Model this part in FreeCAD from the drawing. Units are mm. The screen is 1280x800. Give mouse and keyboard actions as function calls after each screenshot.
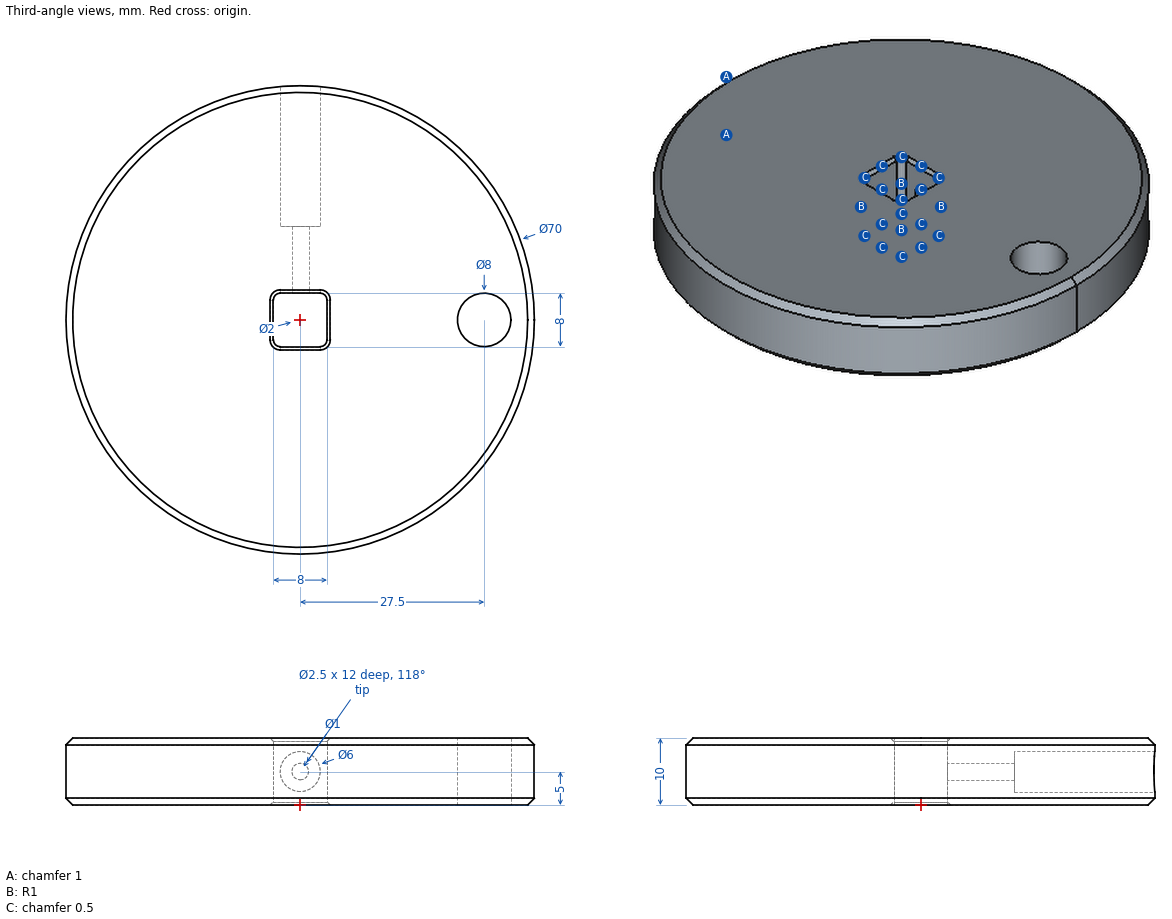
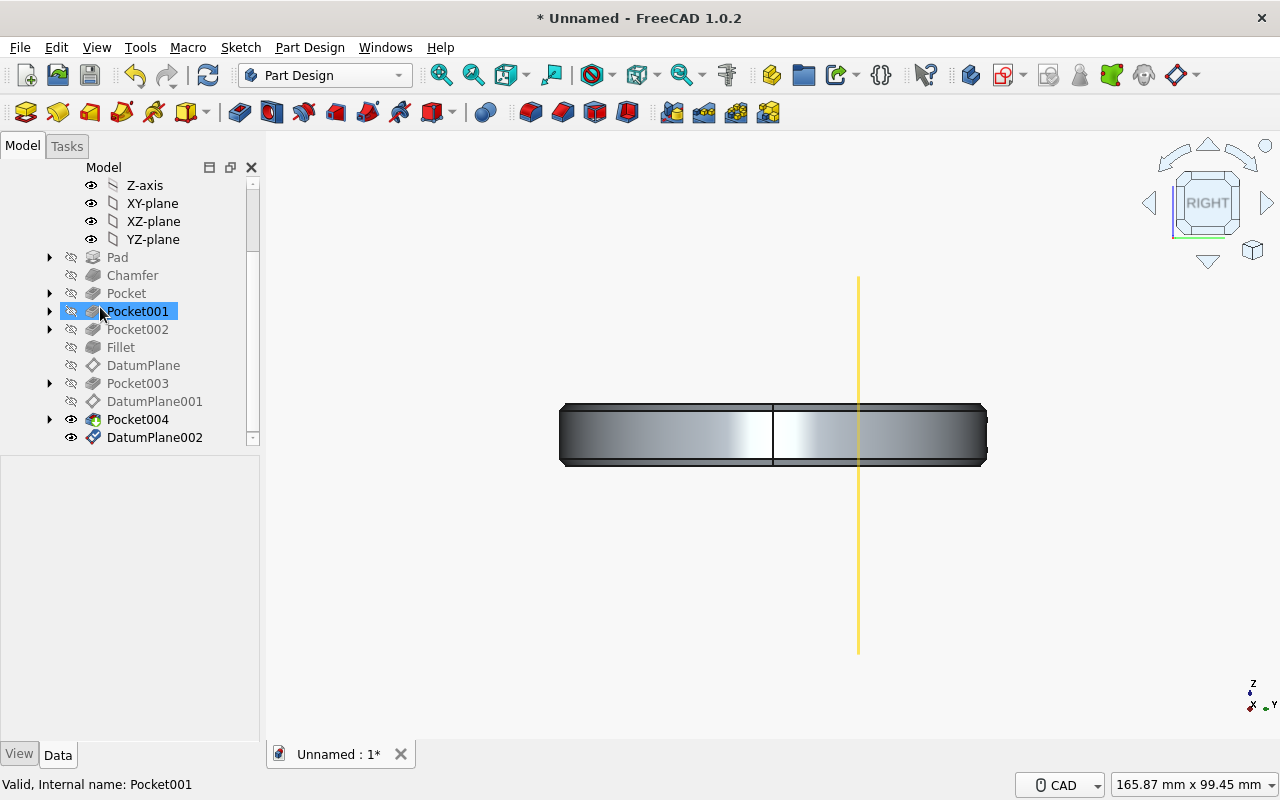
click(116, 437)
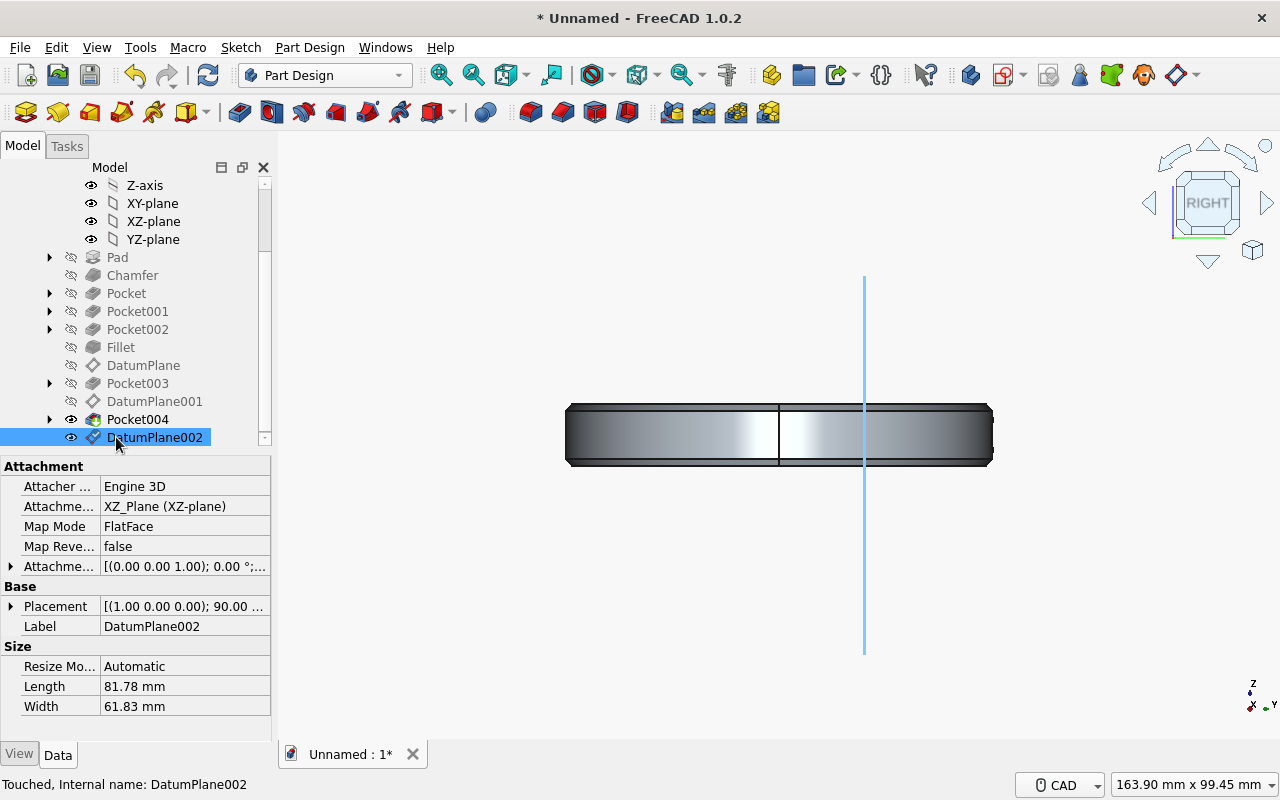
click(1004, 76)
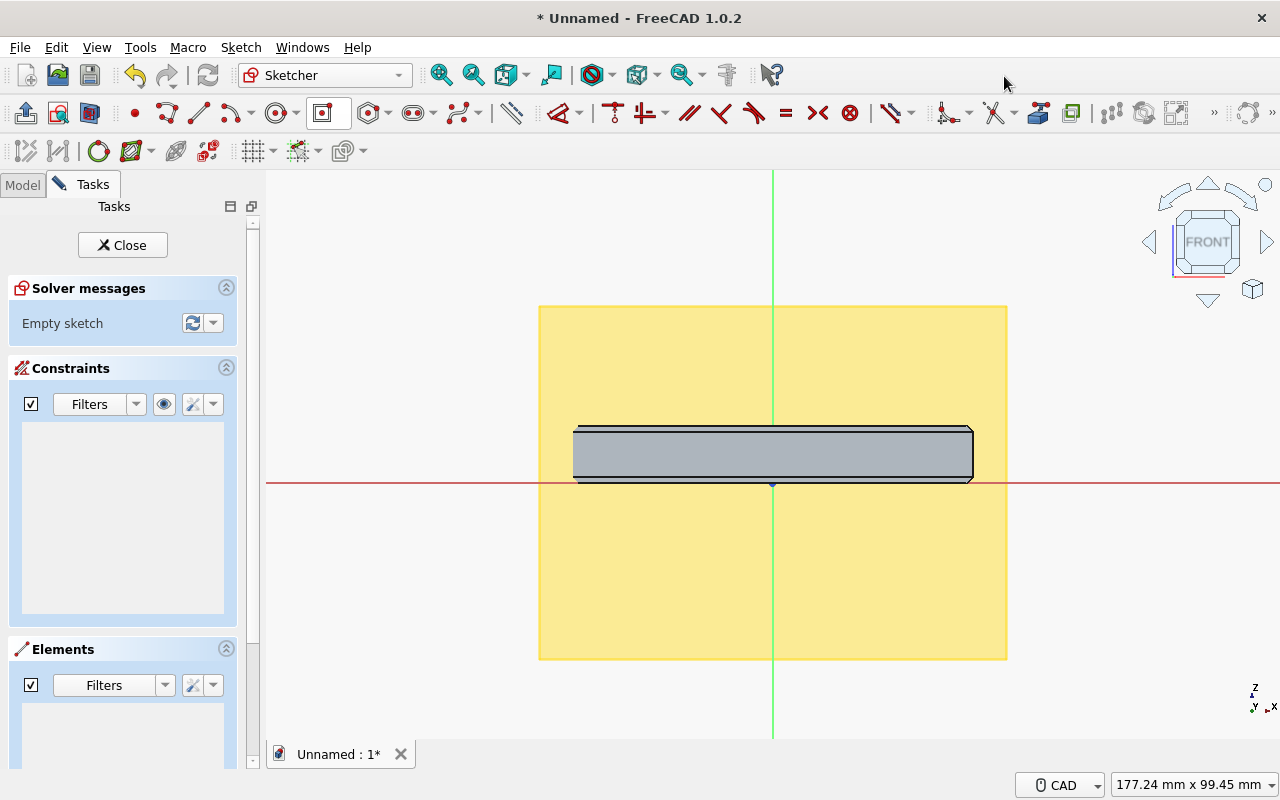
key(q)
key(s)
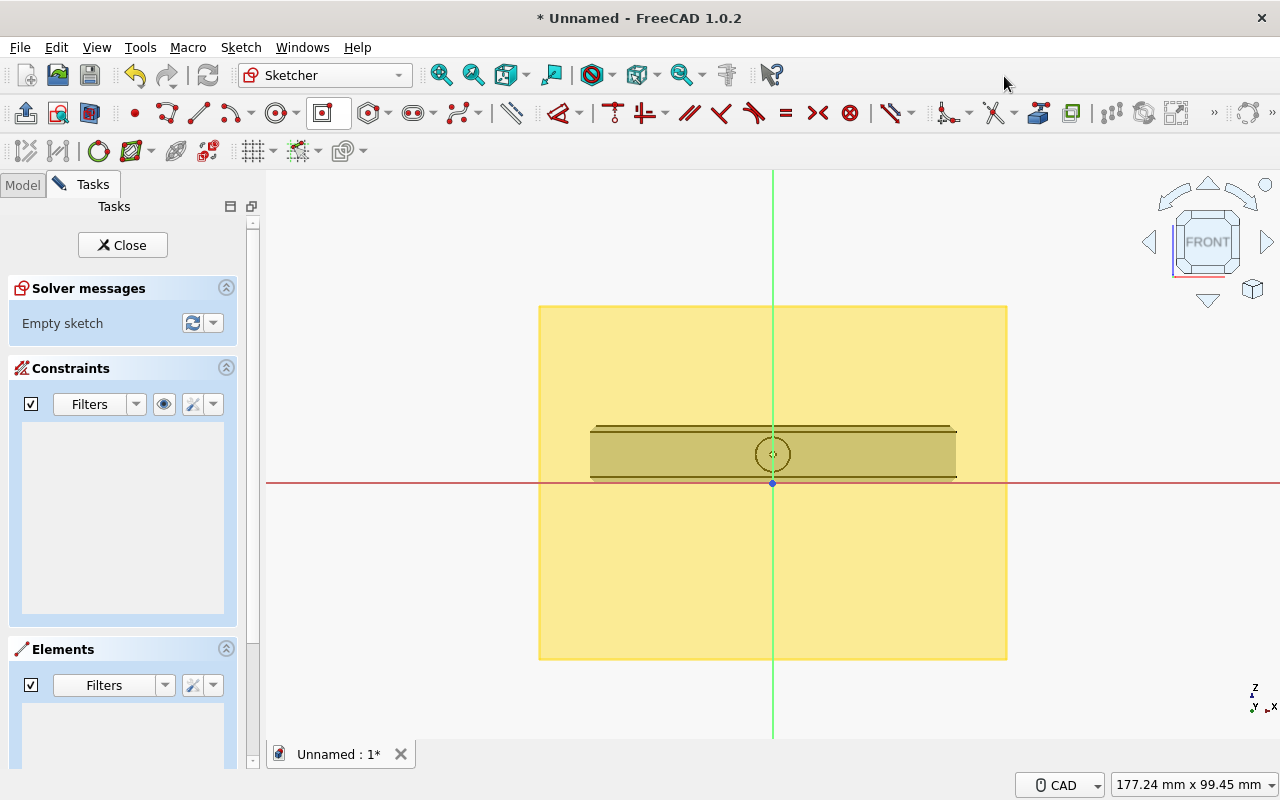
scroll(776, 455, up, 15)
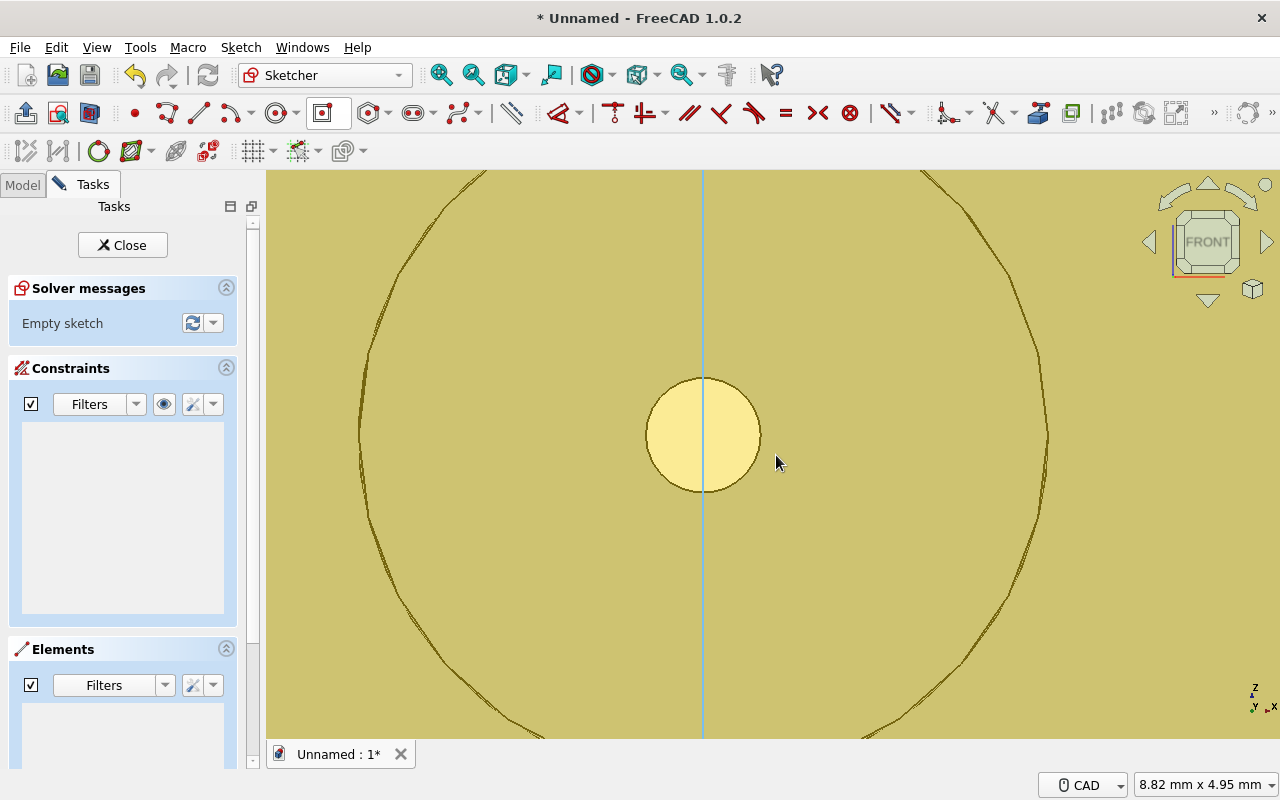
click(276, 114)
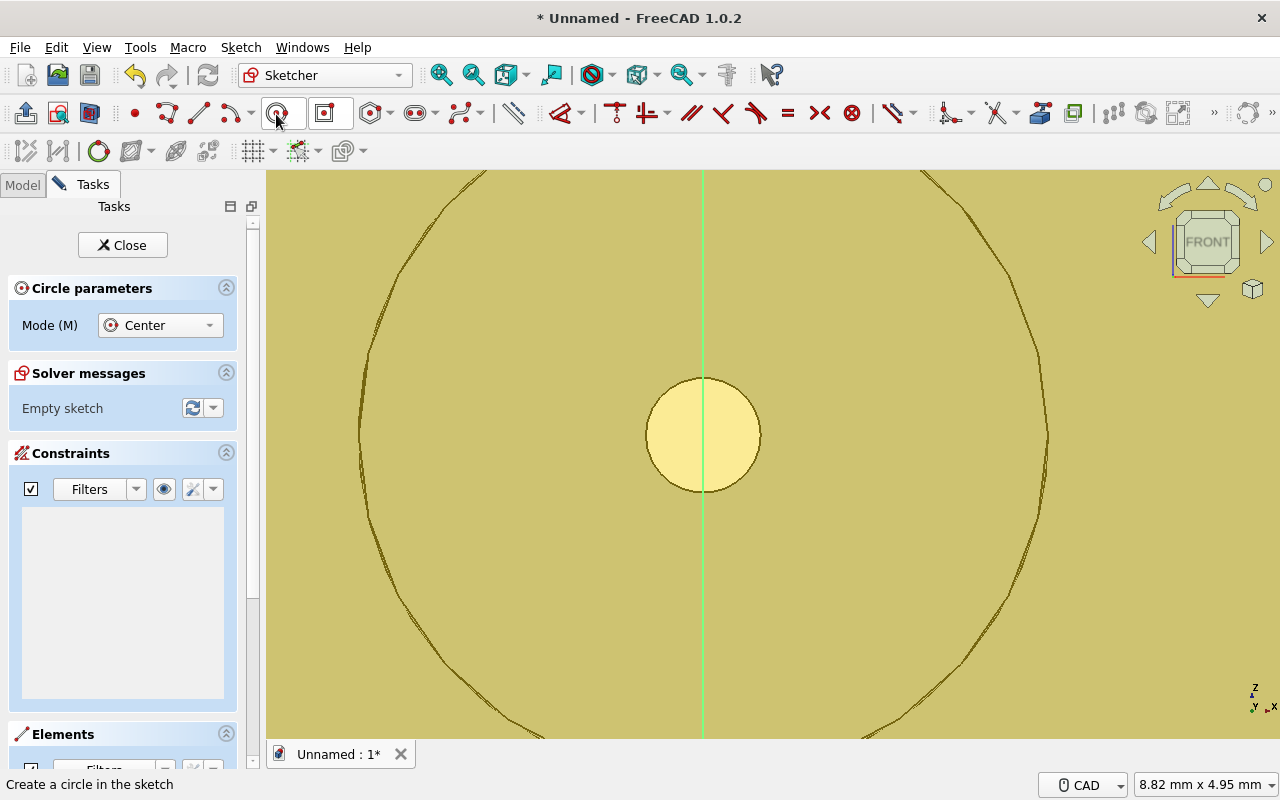
click(703, 435)
click(805, 334)
key(Escape)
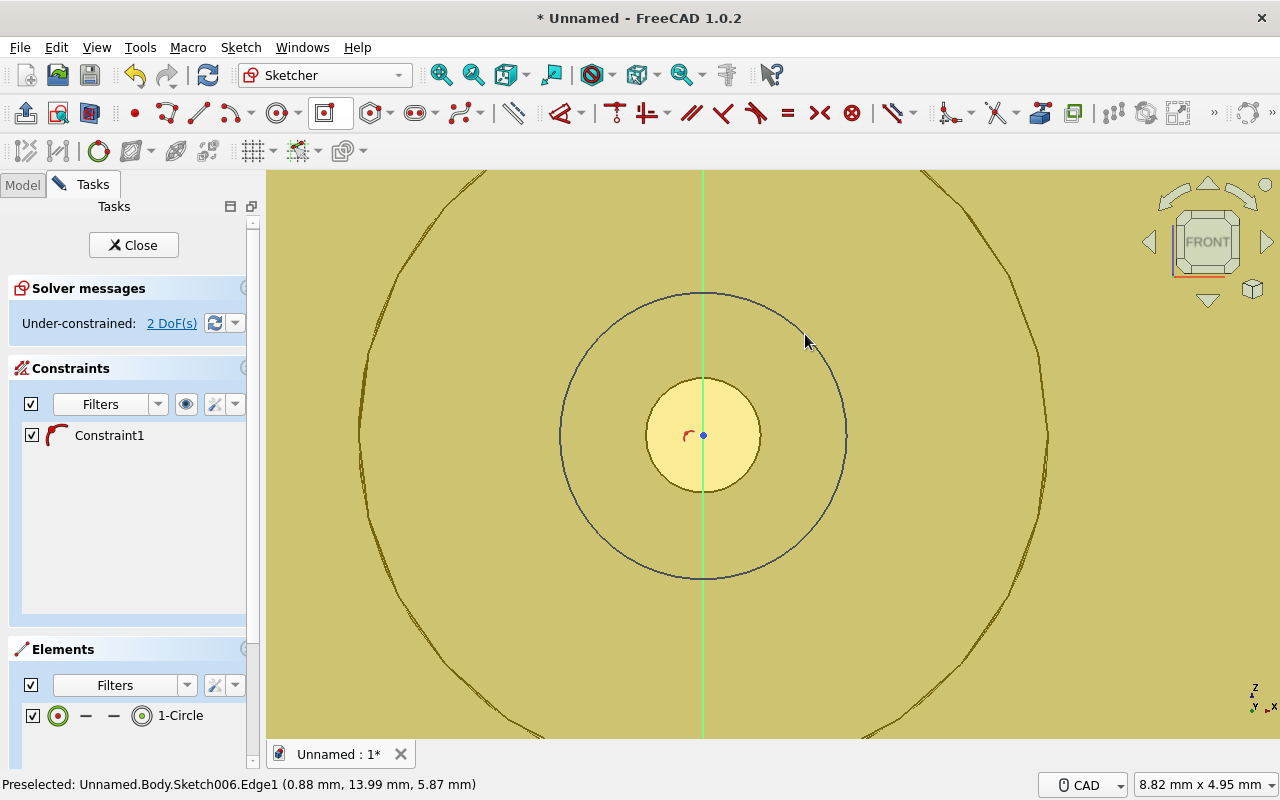
key(d)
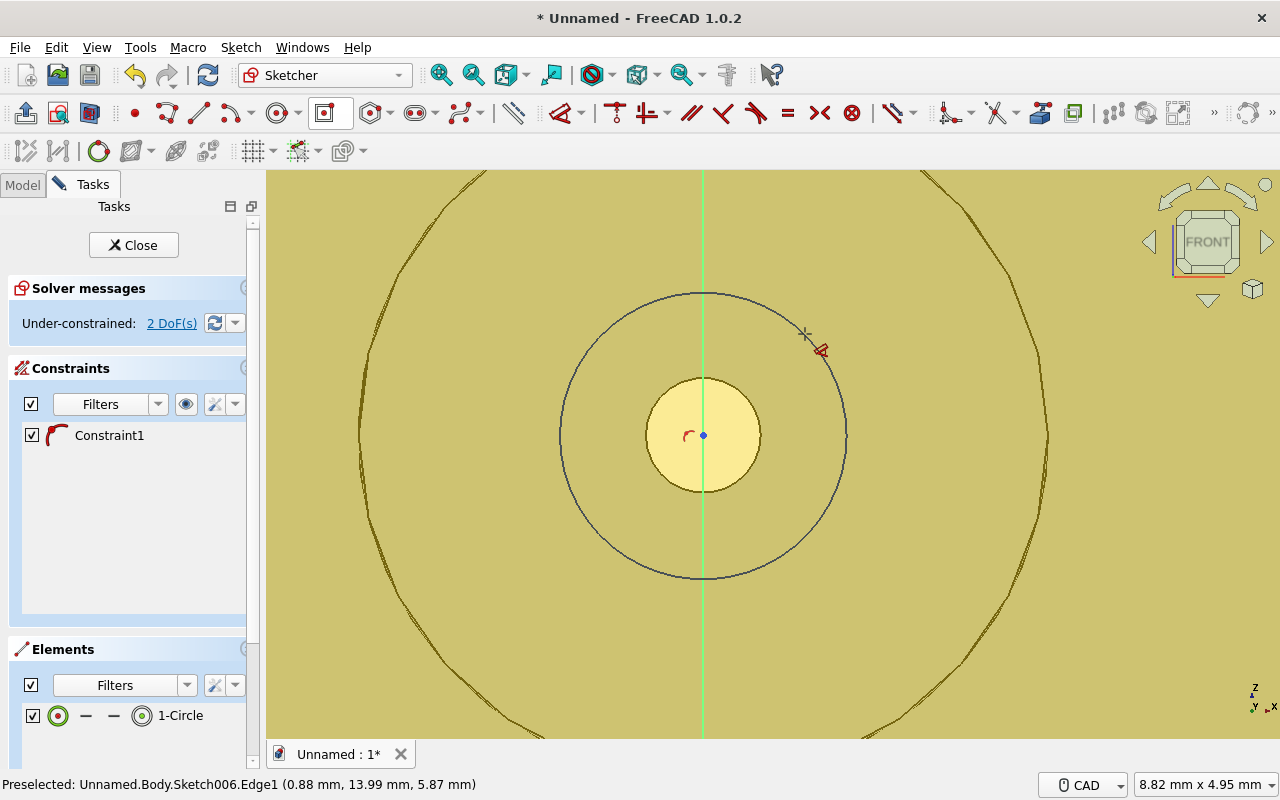
click(804, 334)
click(826, 311)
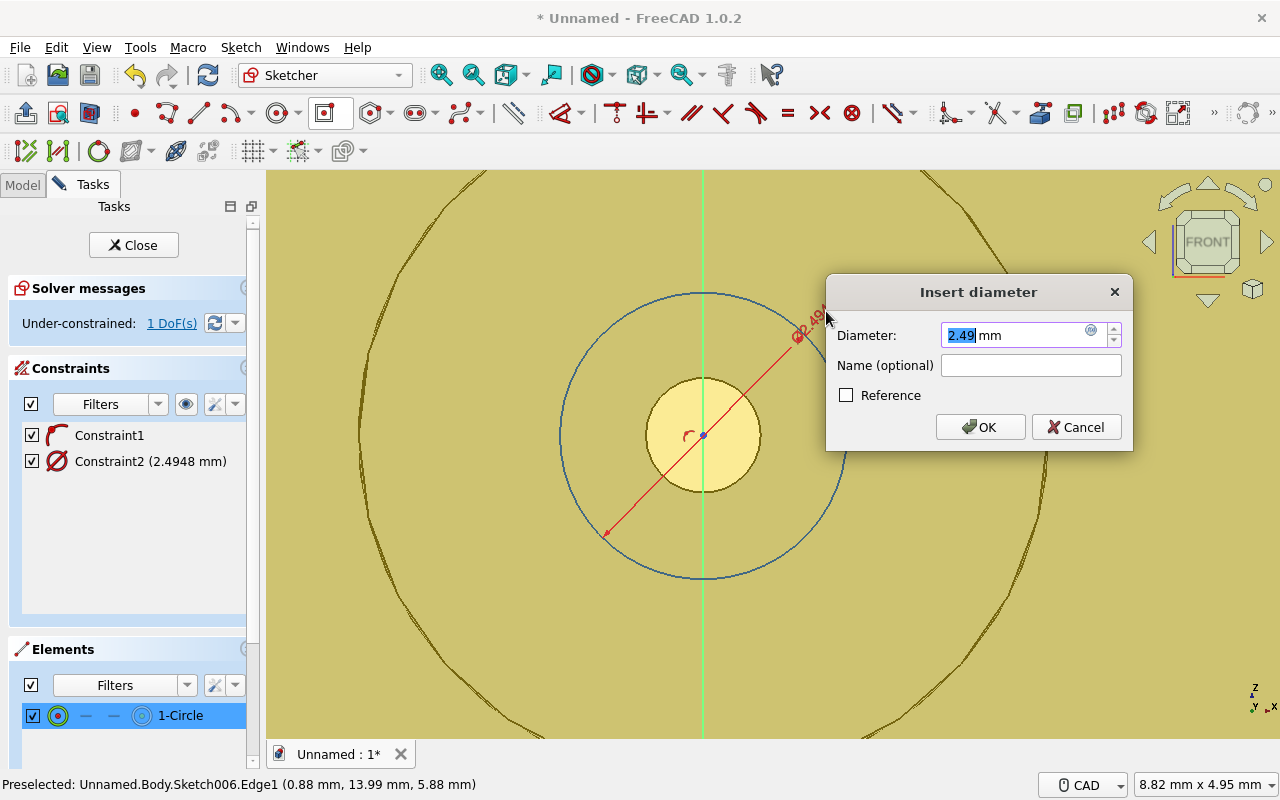
text(2.5)
key(Return)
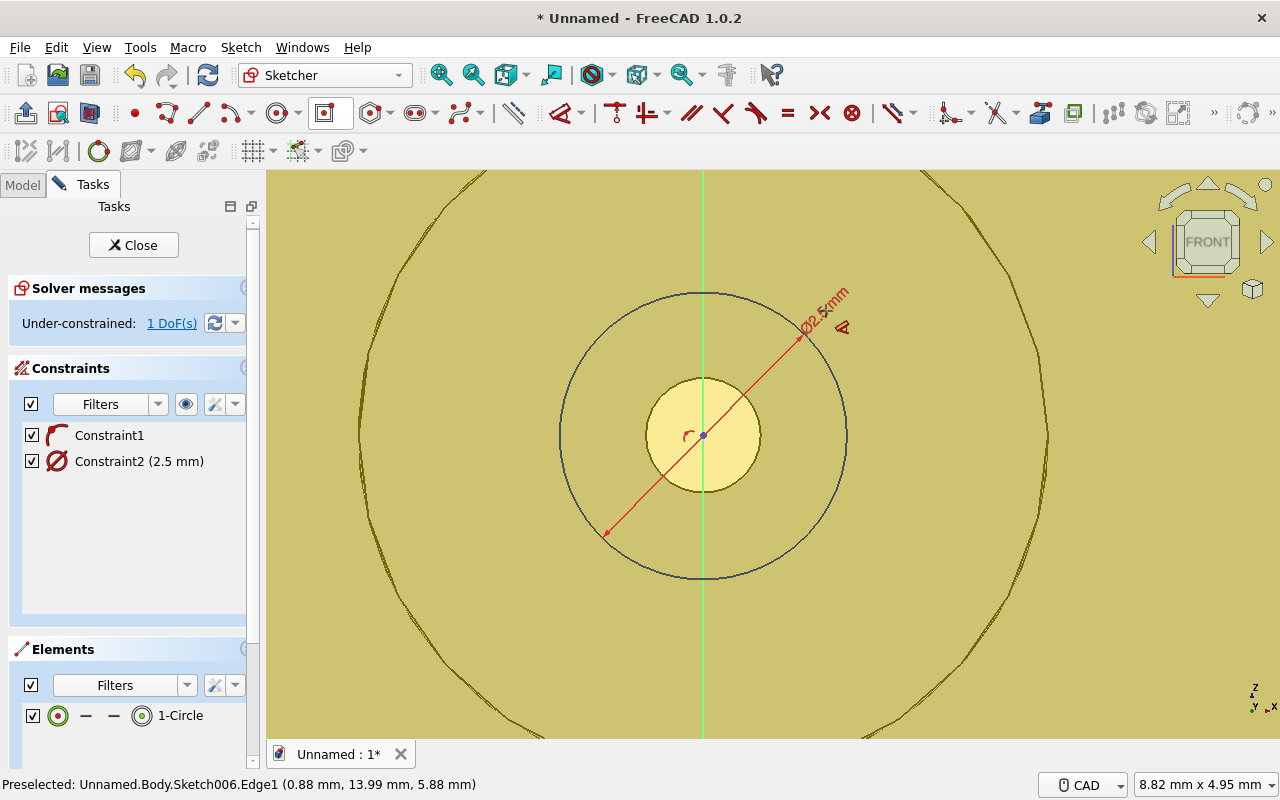
click(703, 436)
click(737, 510)